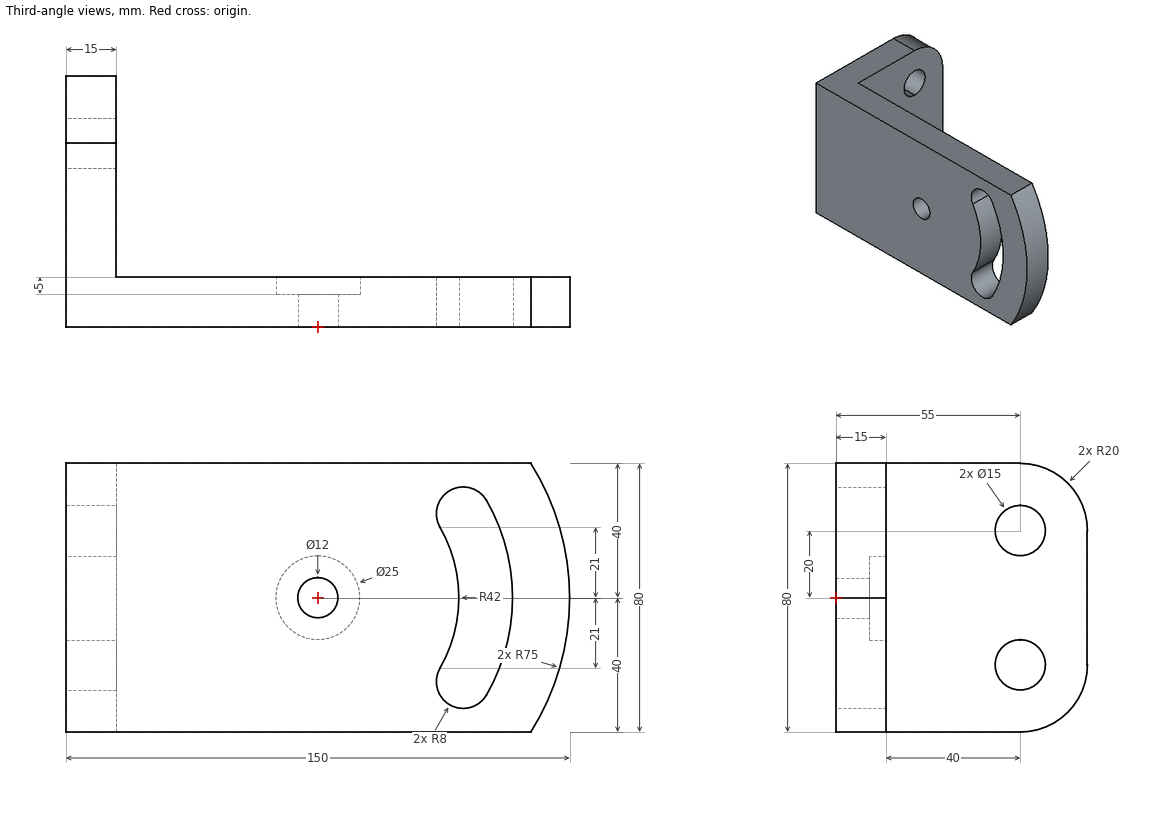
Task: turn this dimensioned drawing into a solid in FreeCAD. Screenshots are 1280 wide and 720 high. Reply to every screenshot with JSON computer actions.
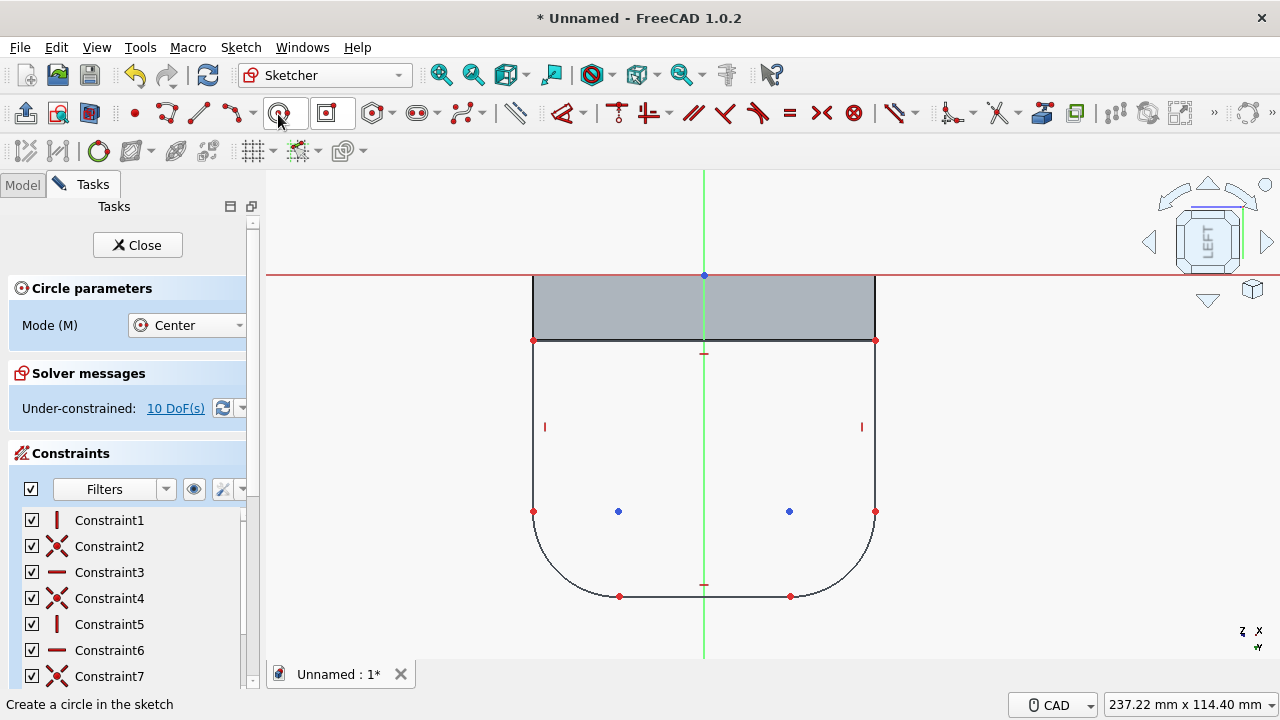
{"action": "left_click", "coordinate": [619, 511]}
{"action": "left_click", "coordinate": [642, 488]}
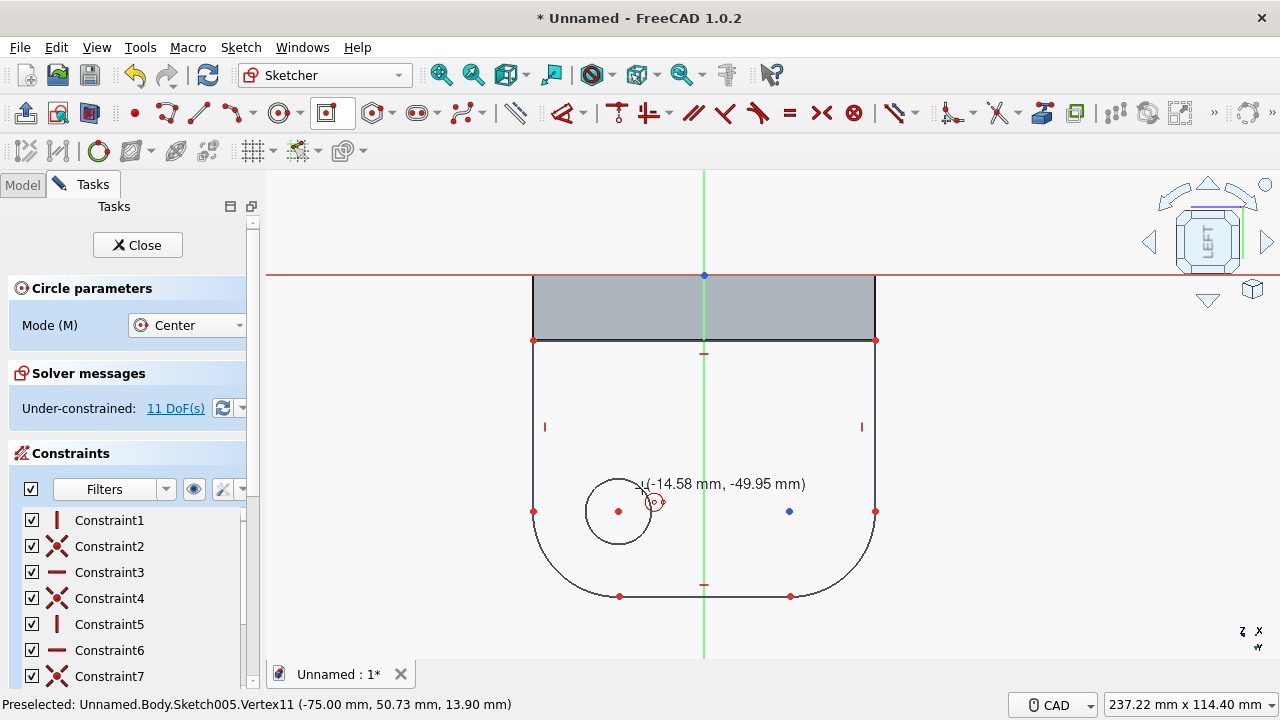
{"action": "left_click", "coordinate": [790, 511]}
{"action": "left_click", "coordinate": [812, 488]}
{"action": "key", "text": "Escape"}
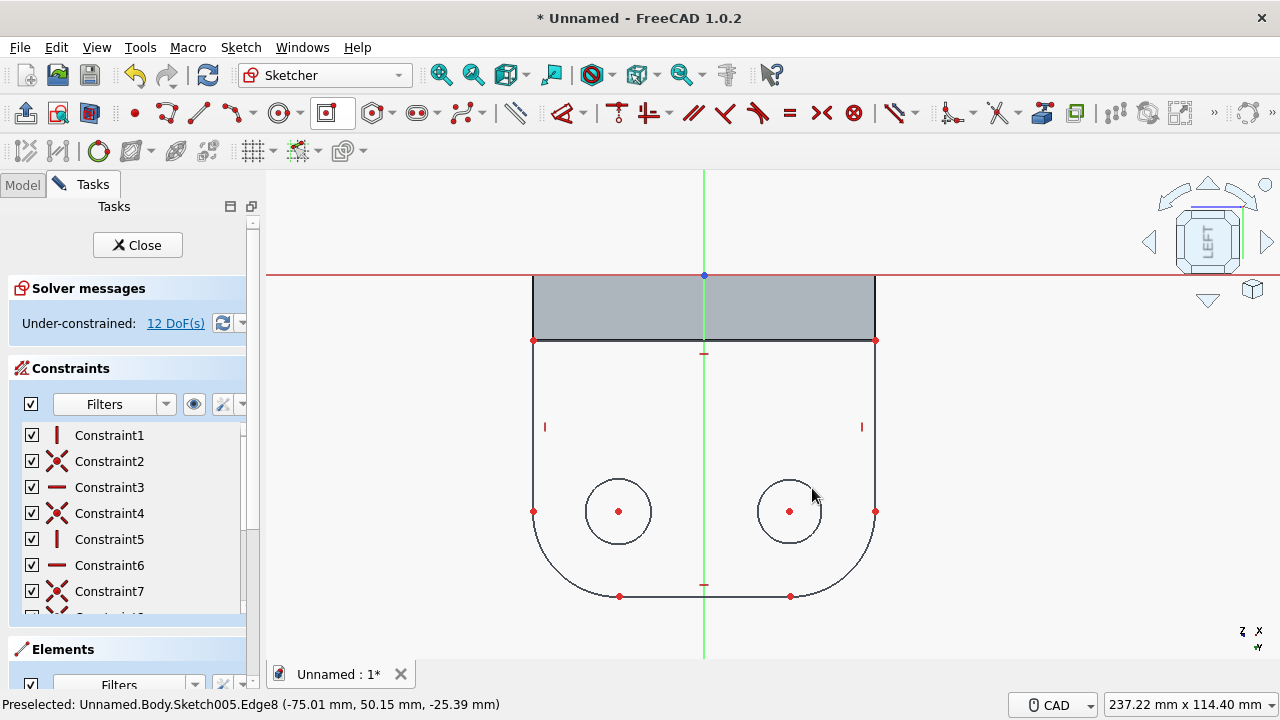
{"action": "left_click", "coordinate": [875, 461]}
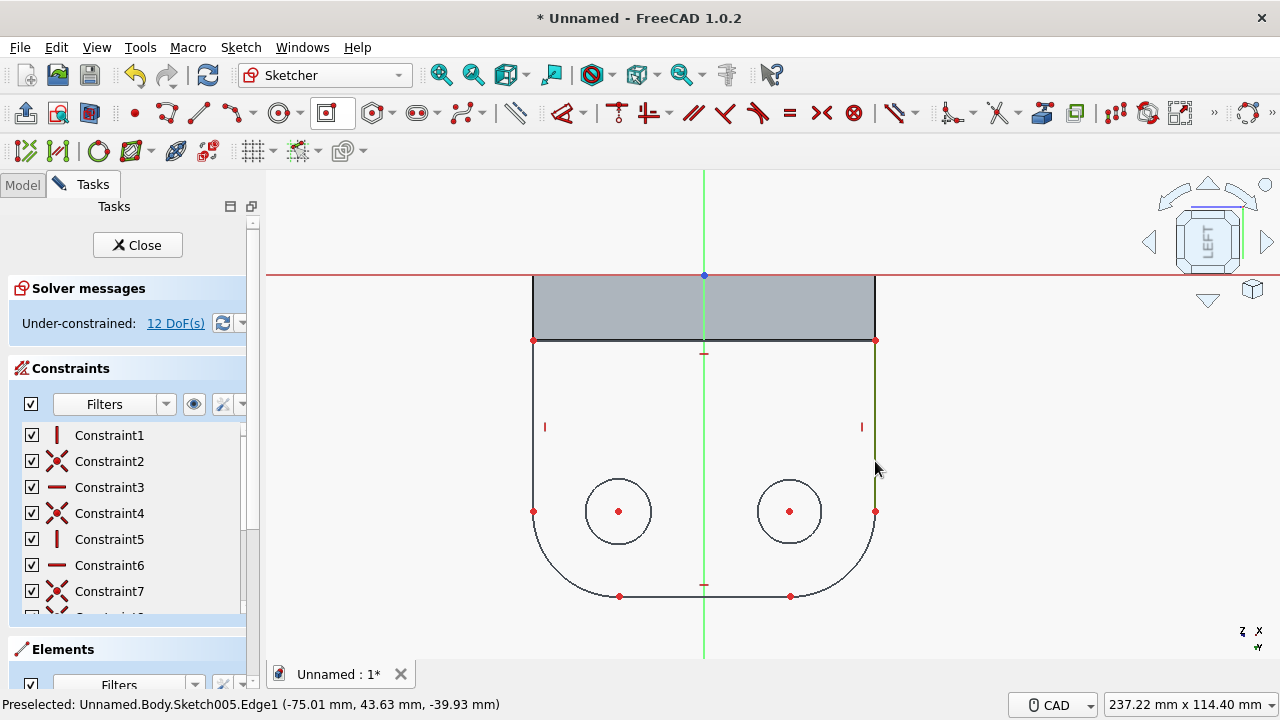
{"action": "left_click", "coordinate": [829, 588]}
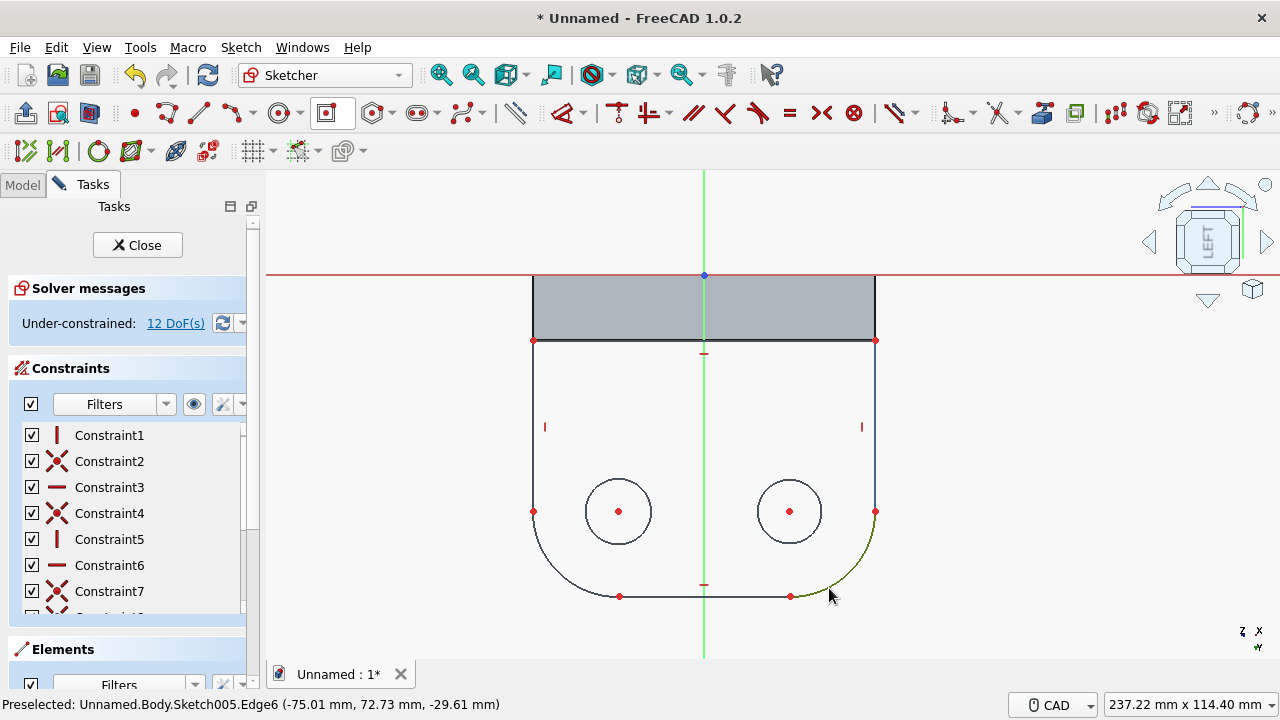
{"action": "key", "text": "t"}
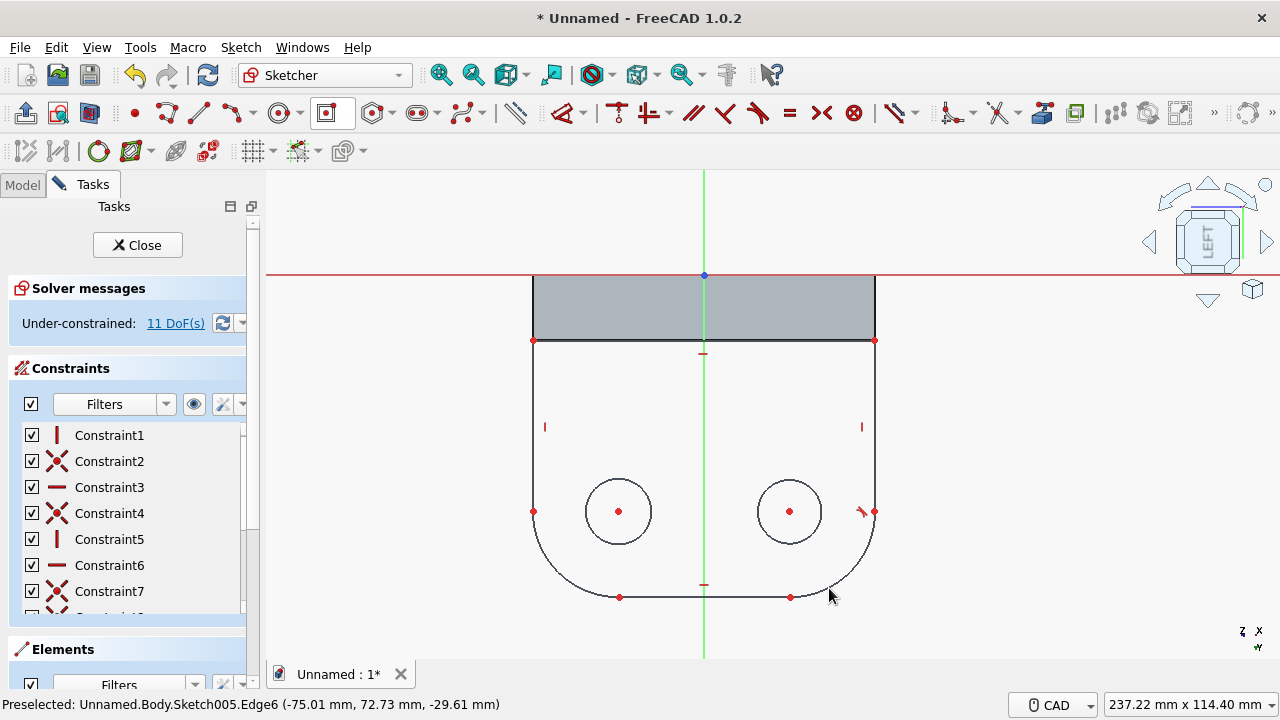
{"action": "left_click", "coordinate": [533, 392]}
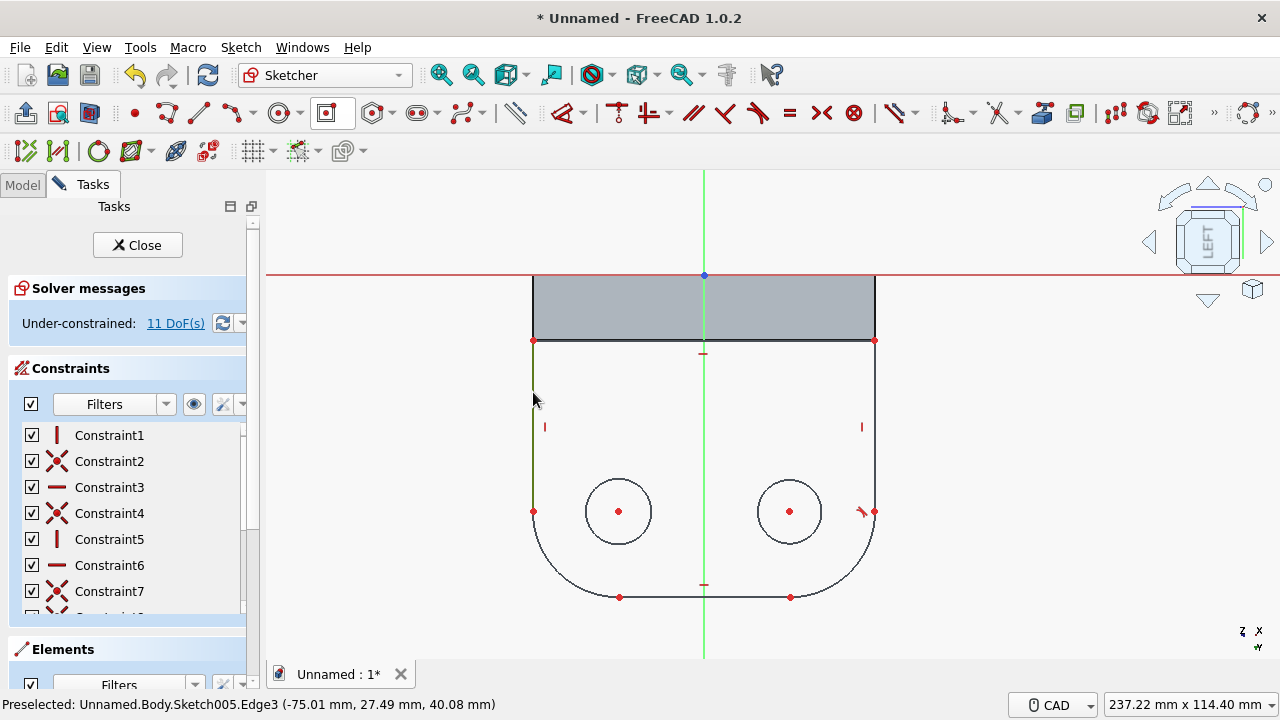
{"action": "left_click", "coordinate": [542, 551]}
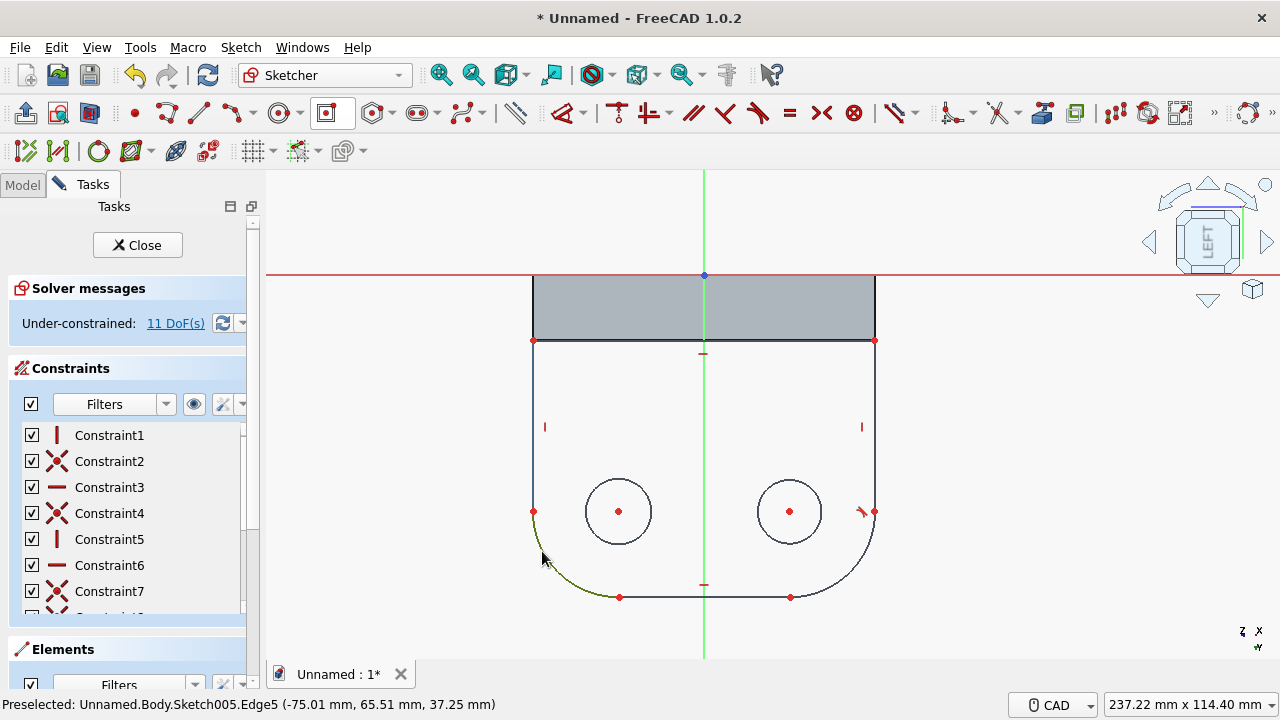
{"action": "left_click", "coordinate": [758, 114]}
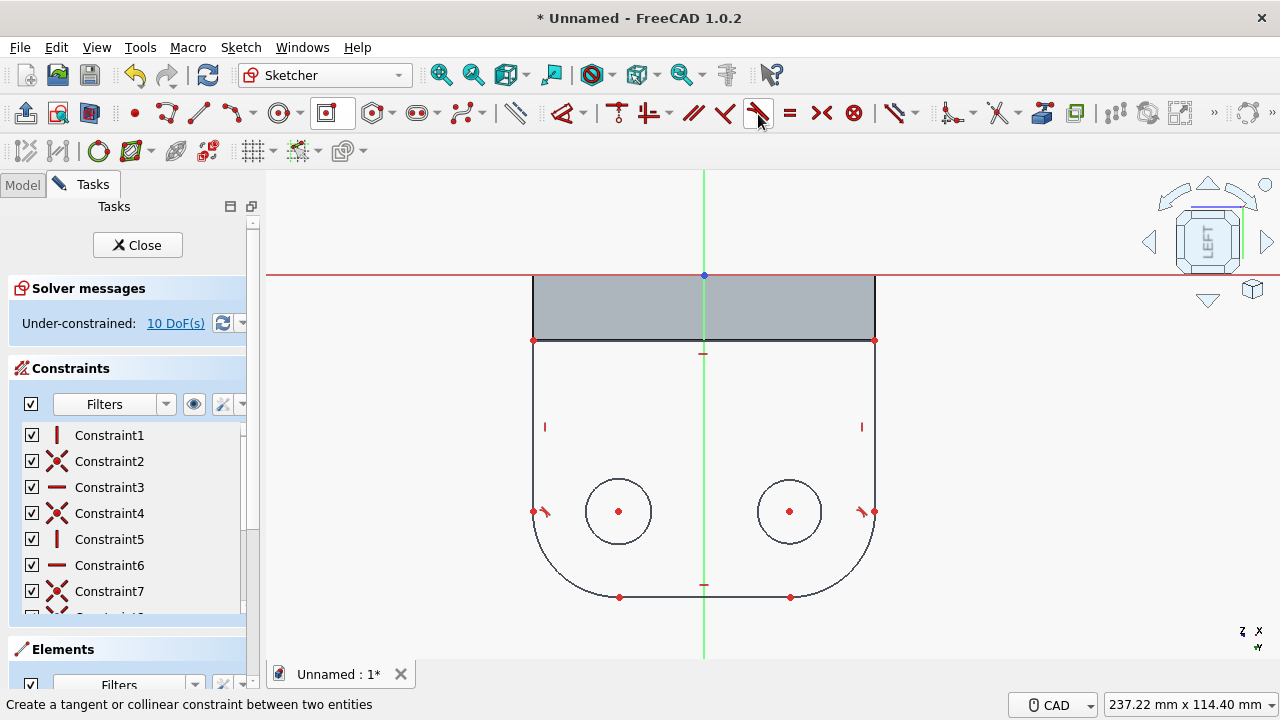
{"action": "left_click", "coordinate": [670, 597]}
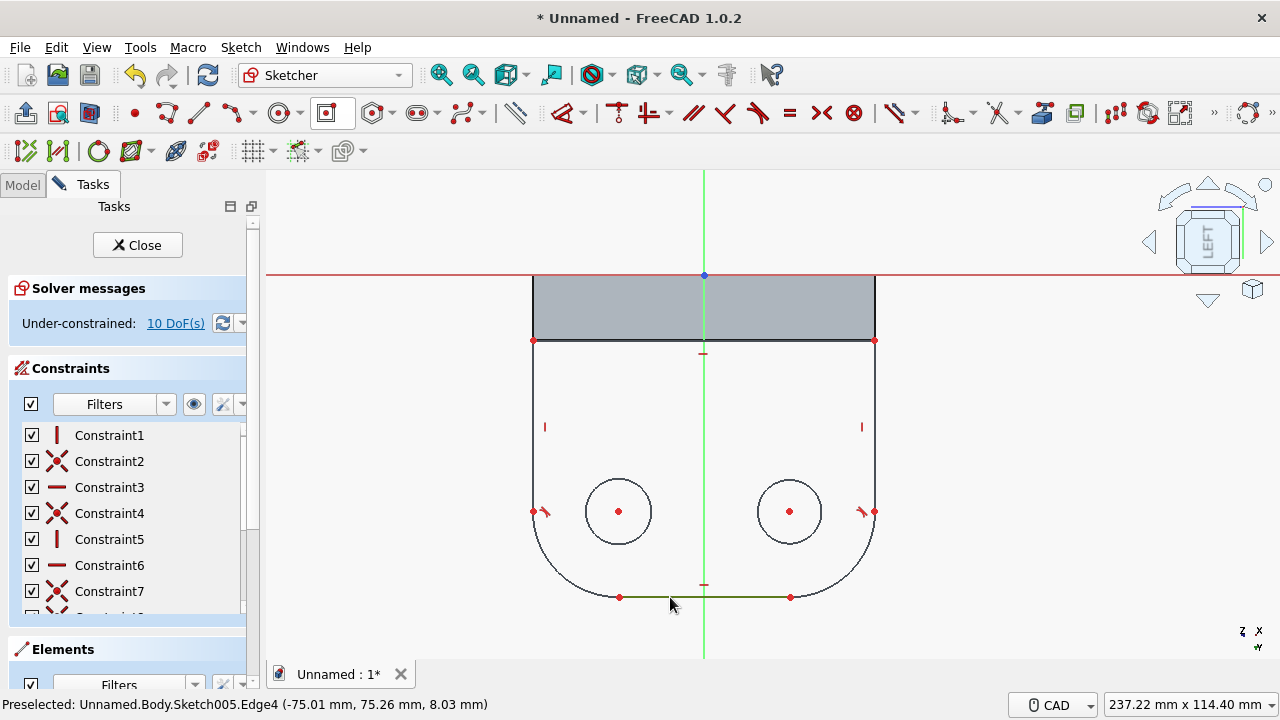
{"action": "left_click", "coordinate": [542, 551]}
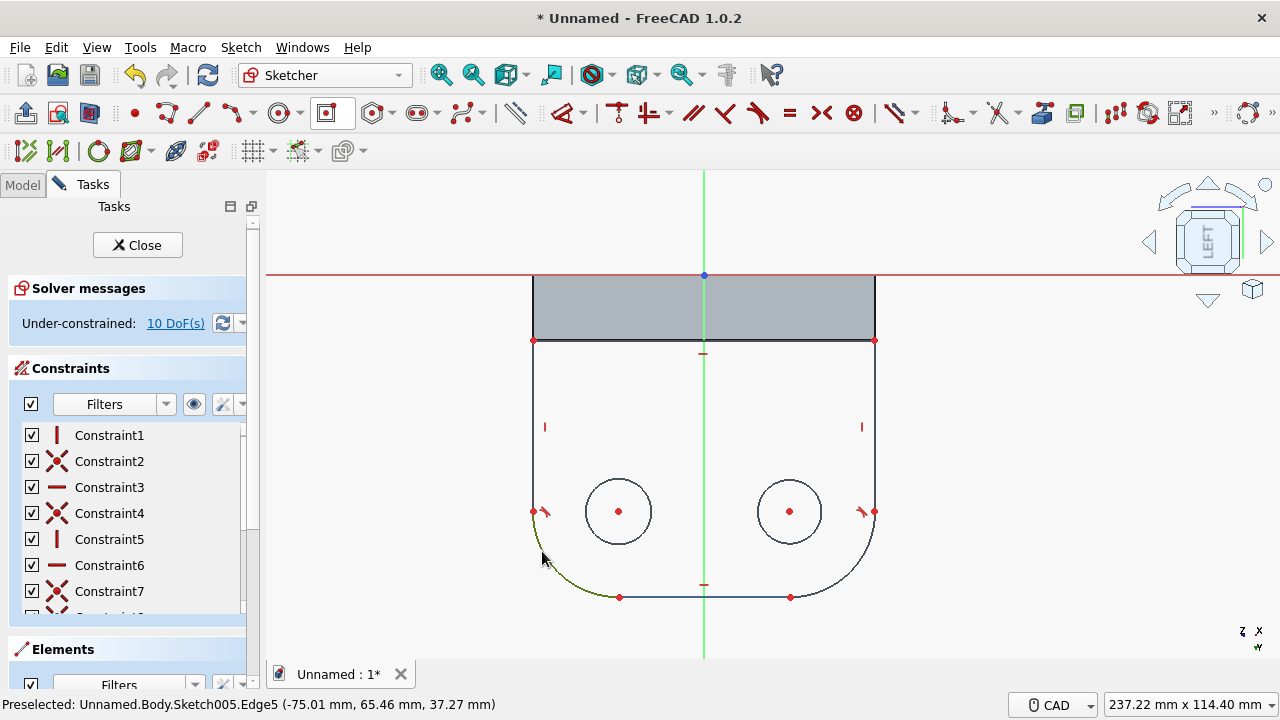
{"action": "key", "text": "t"}